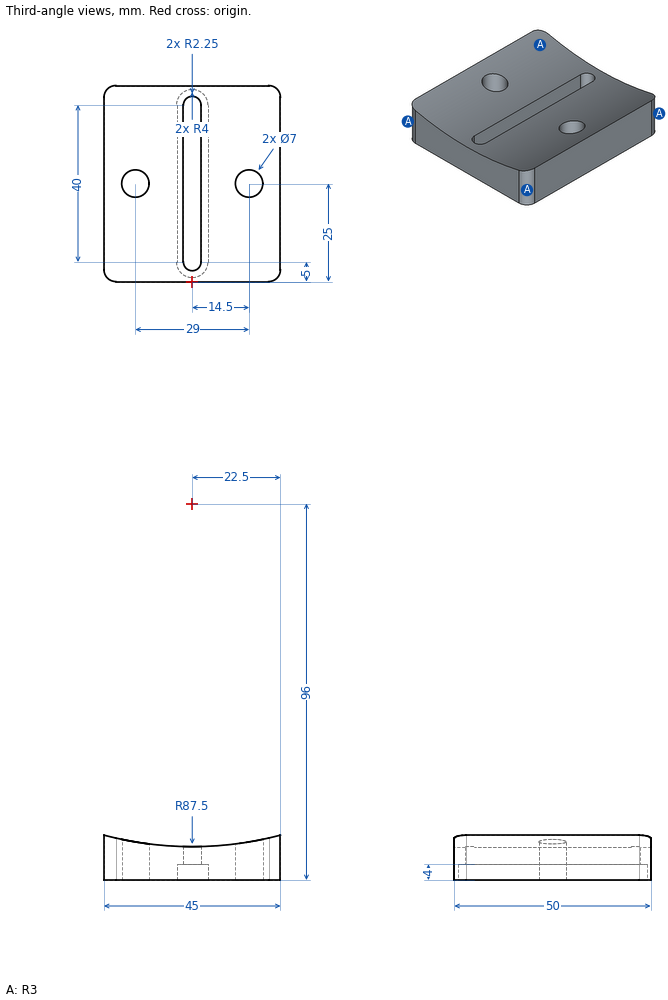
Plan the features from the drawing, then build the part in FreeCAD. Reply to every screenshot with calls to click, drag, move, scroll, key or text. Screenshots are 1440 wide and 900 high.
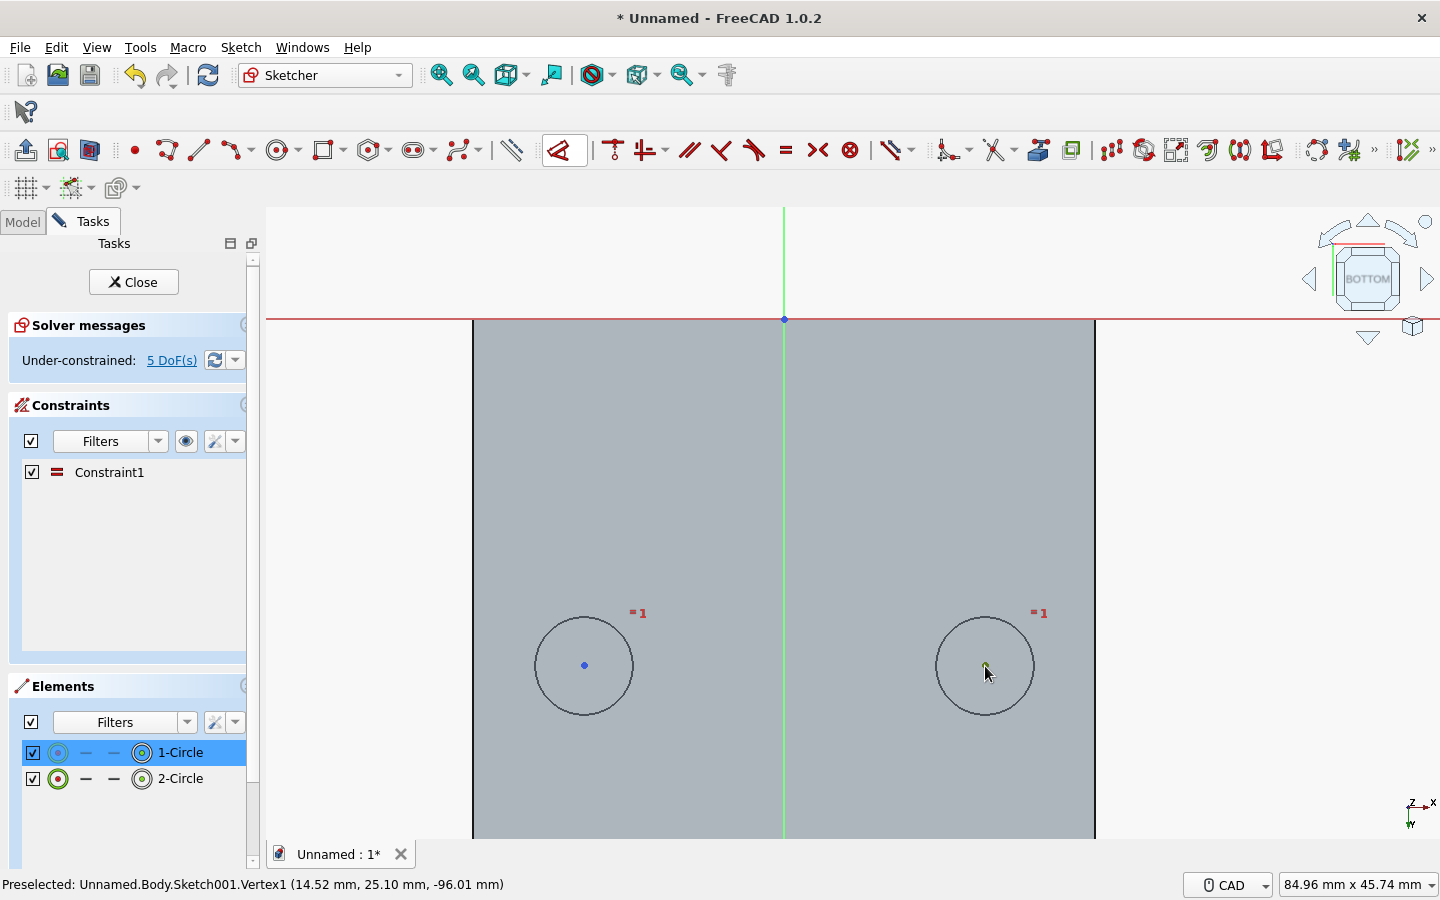
click(584, 666)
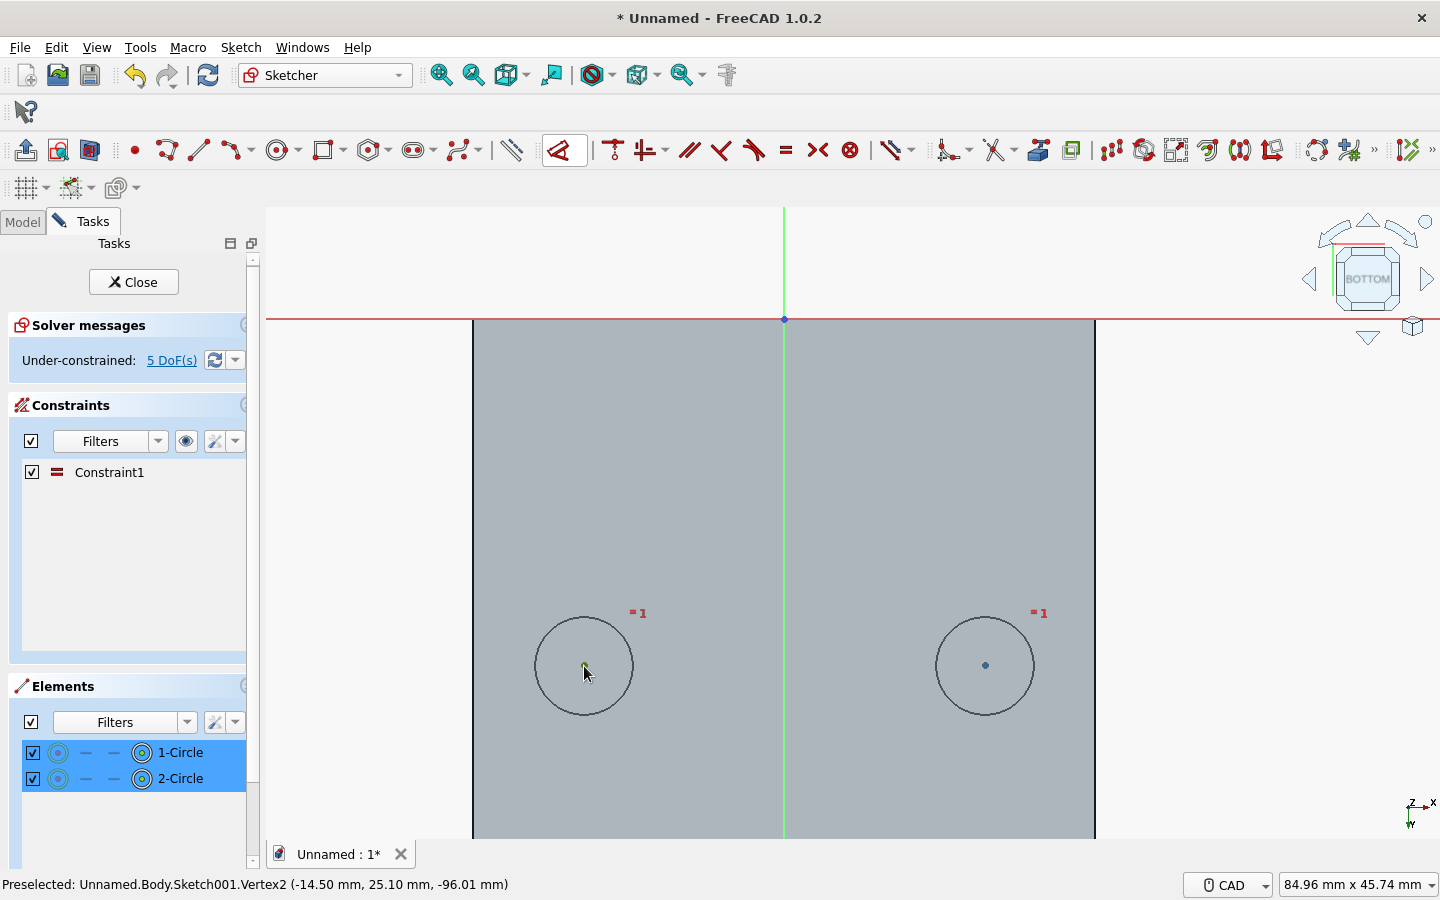
click(668, 150)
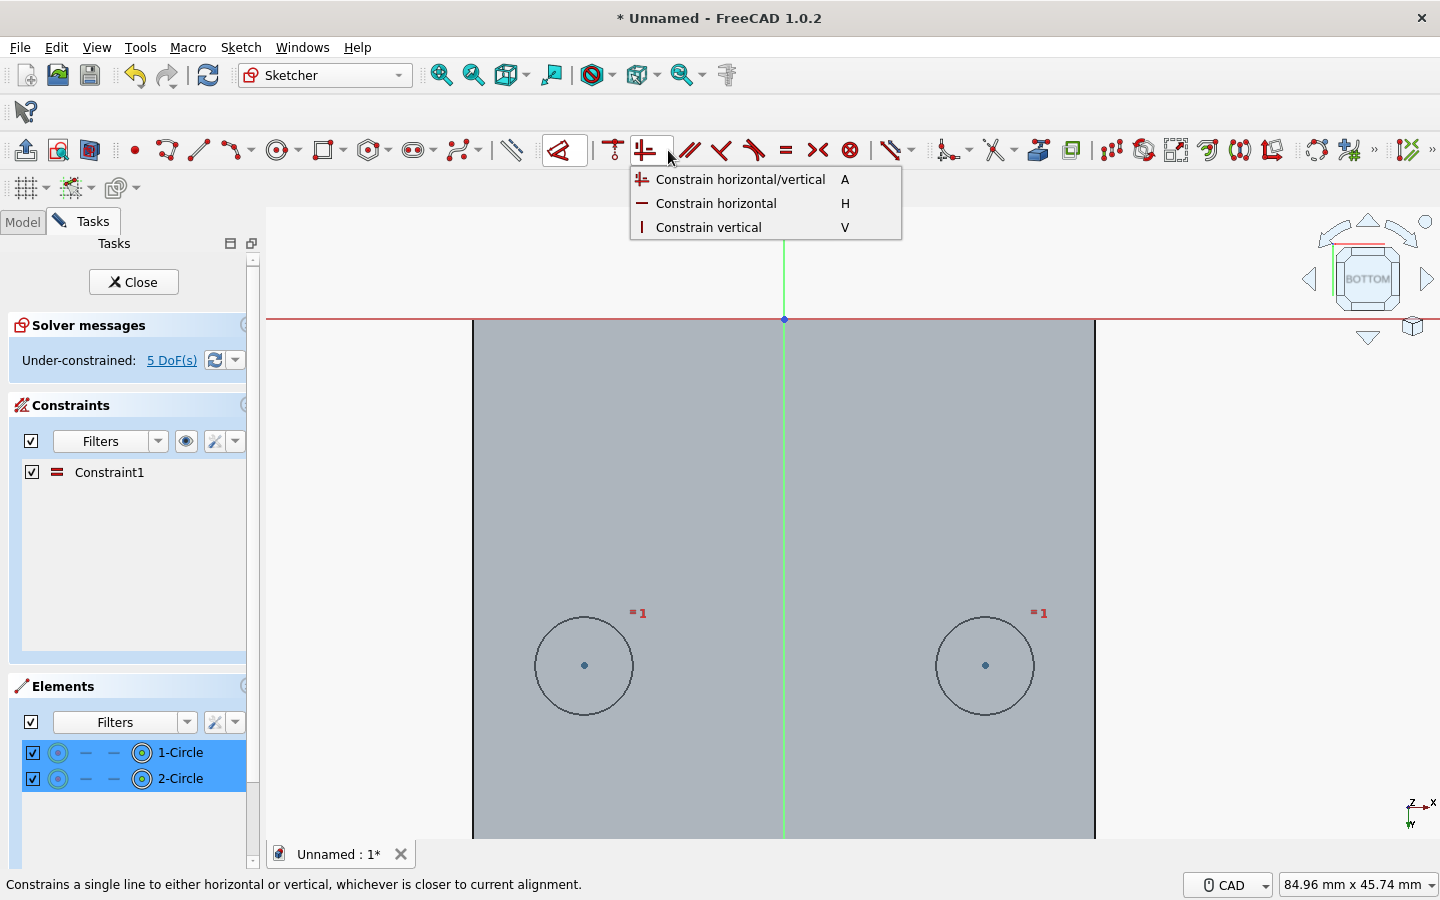
click(766, 203)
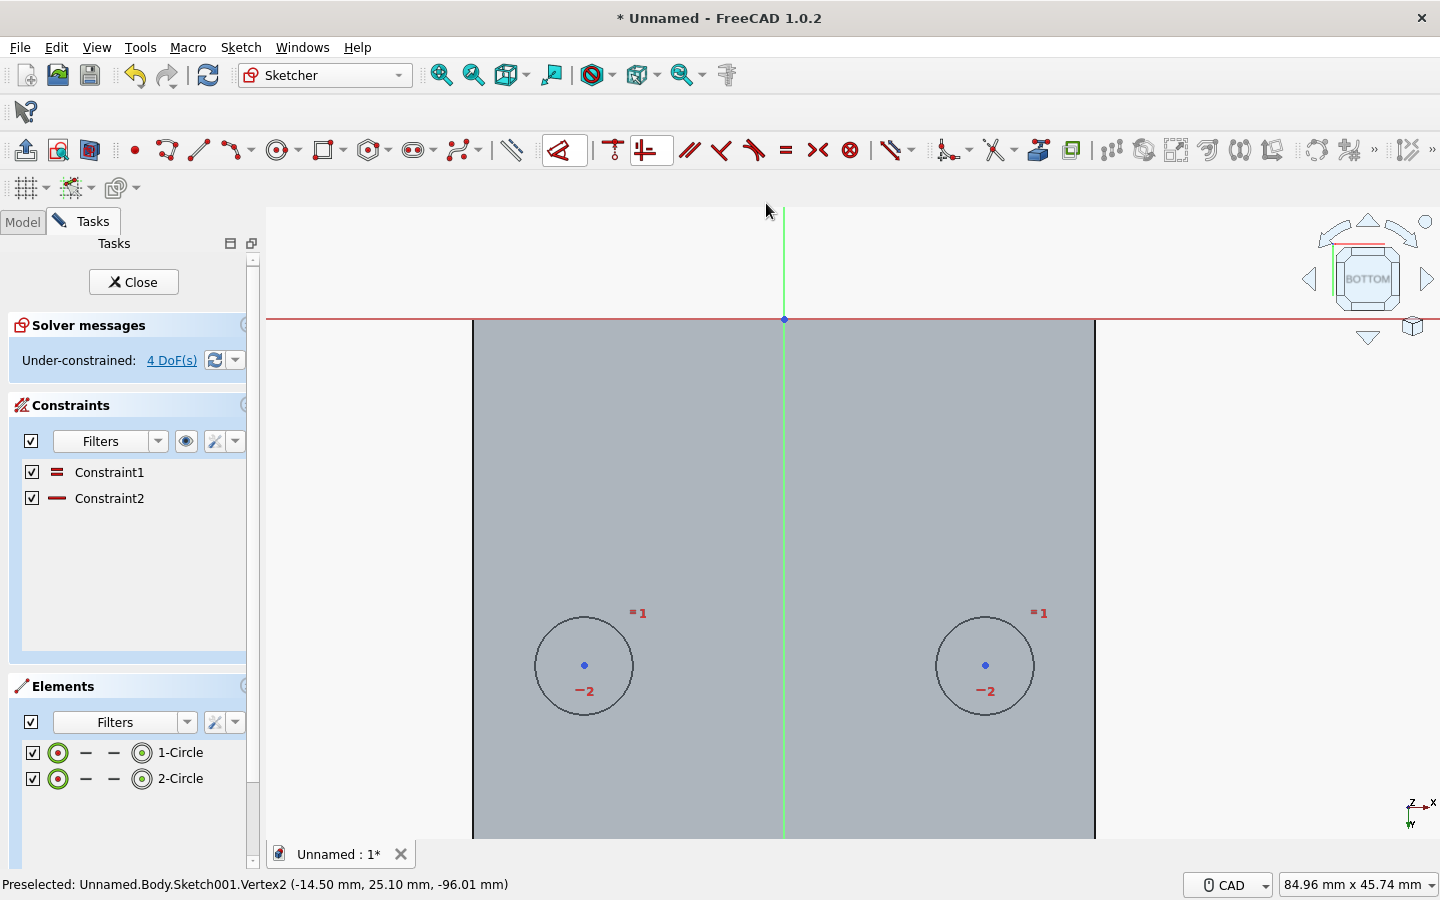
click(558, 150)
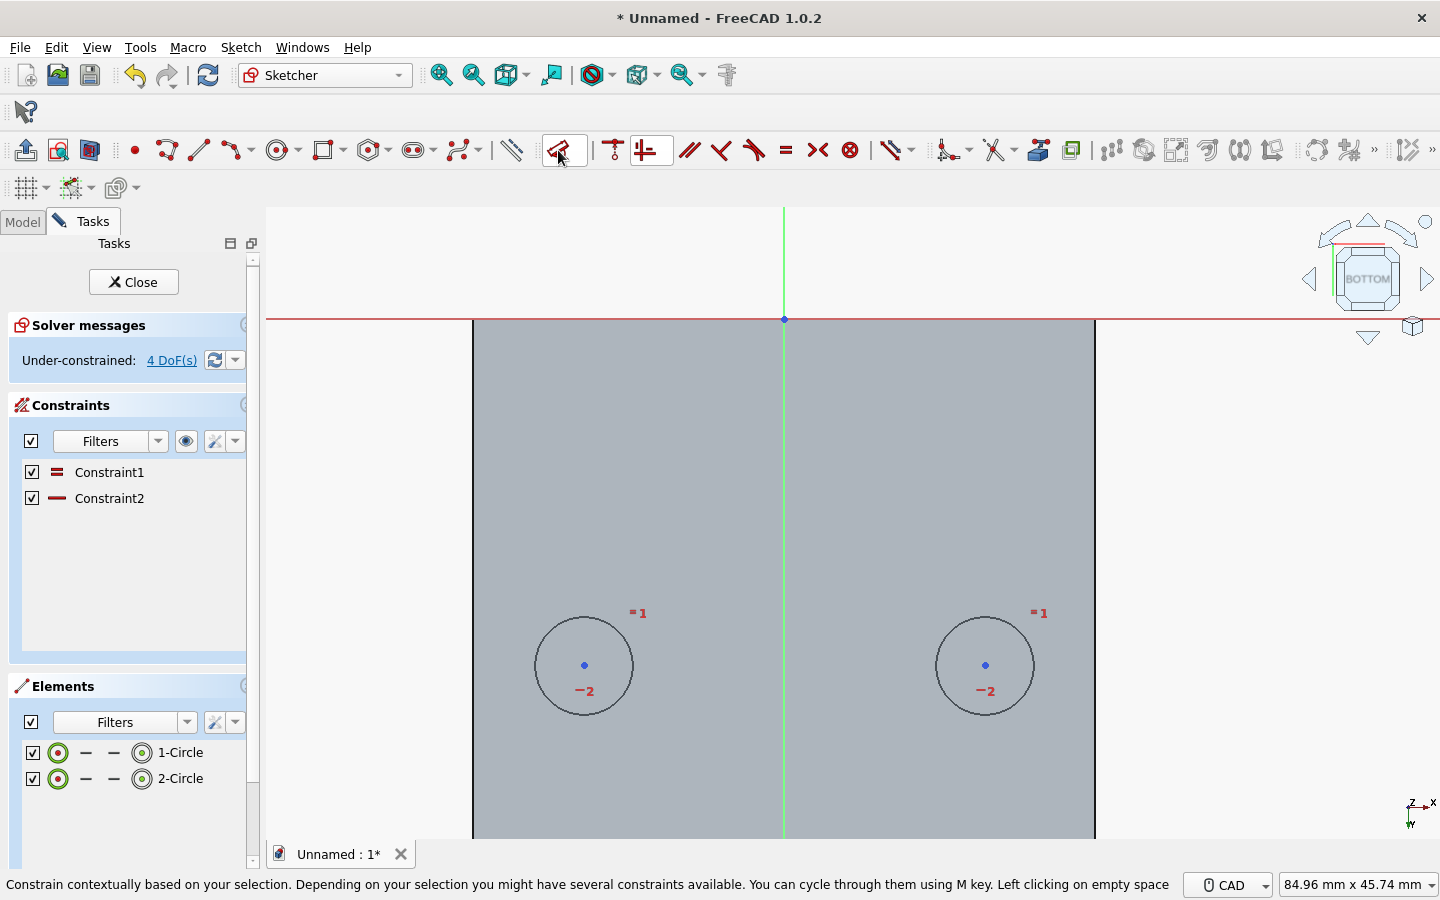
click(1019, 631)
click(1041, 608)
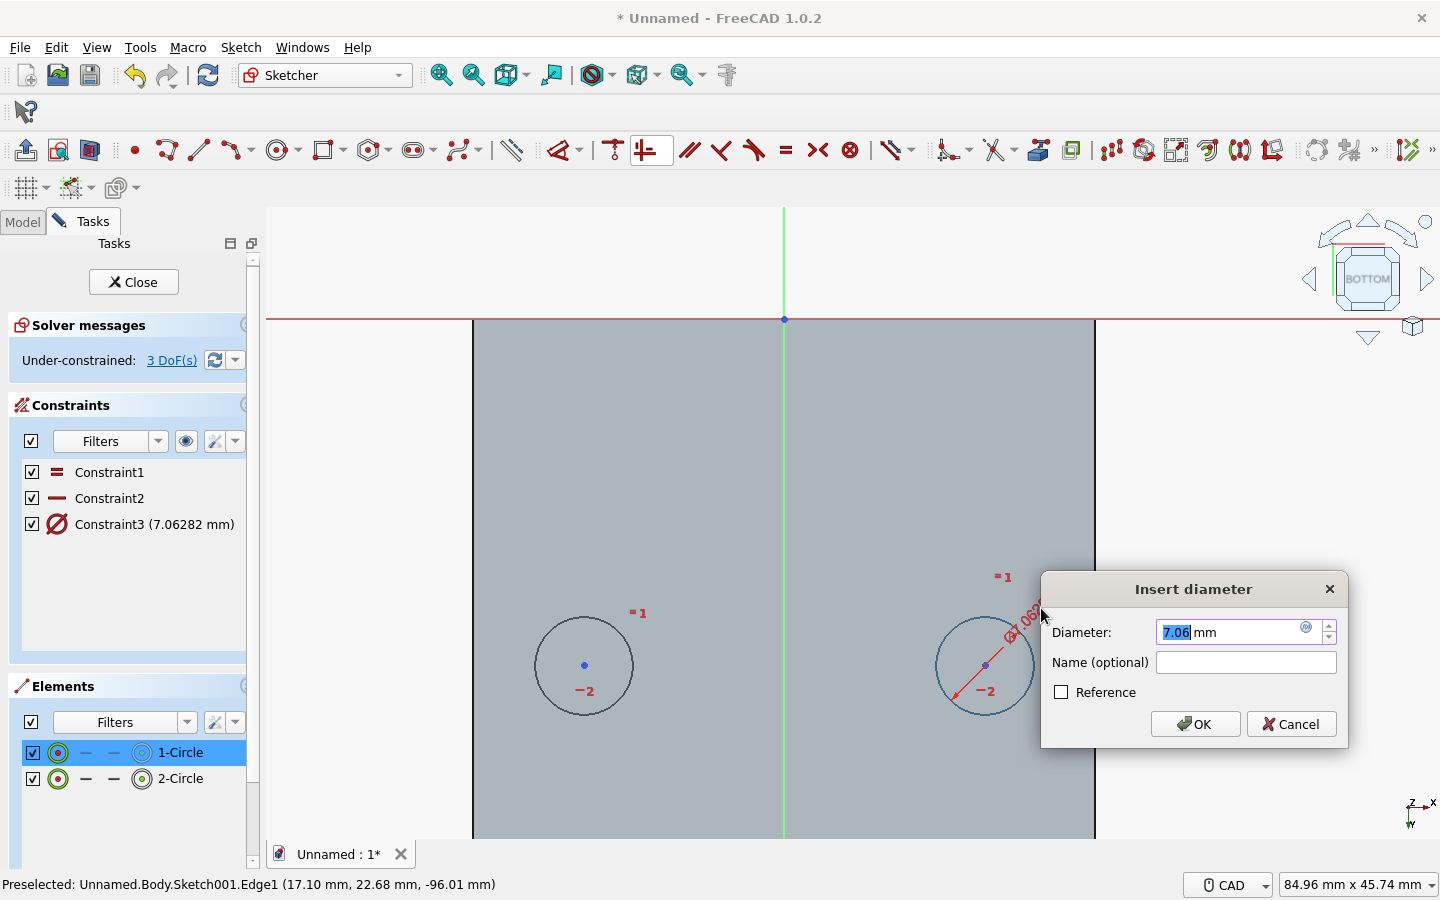
text(7)
key(Return)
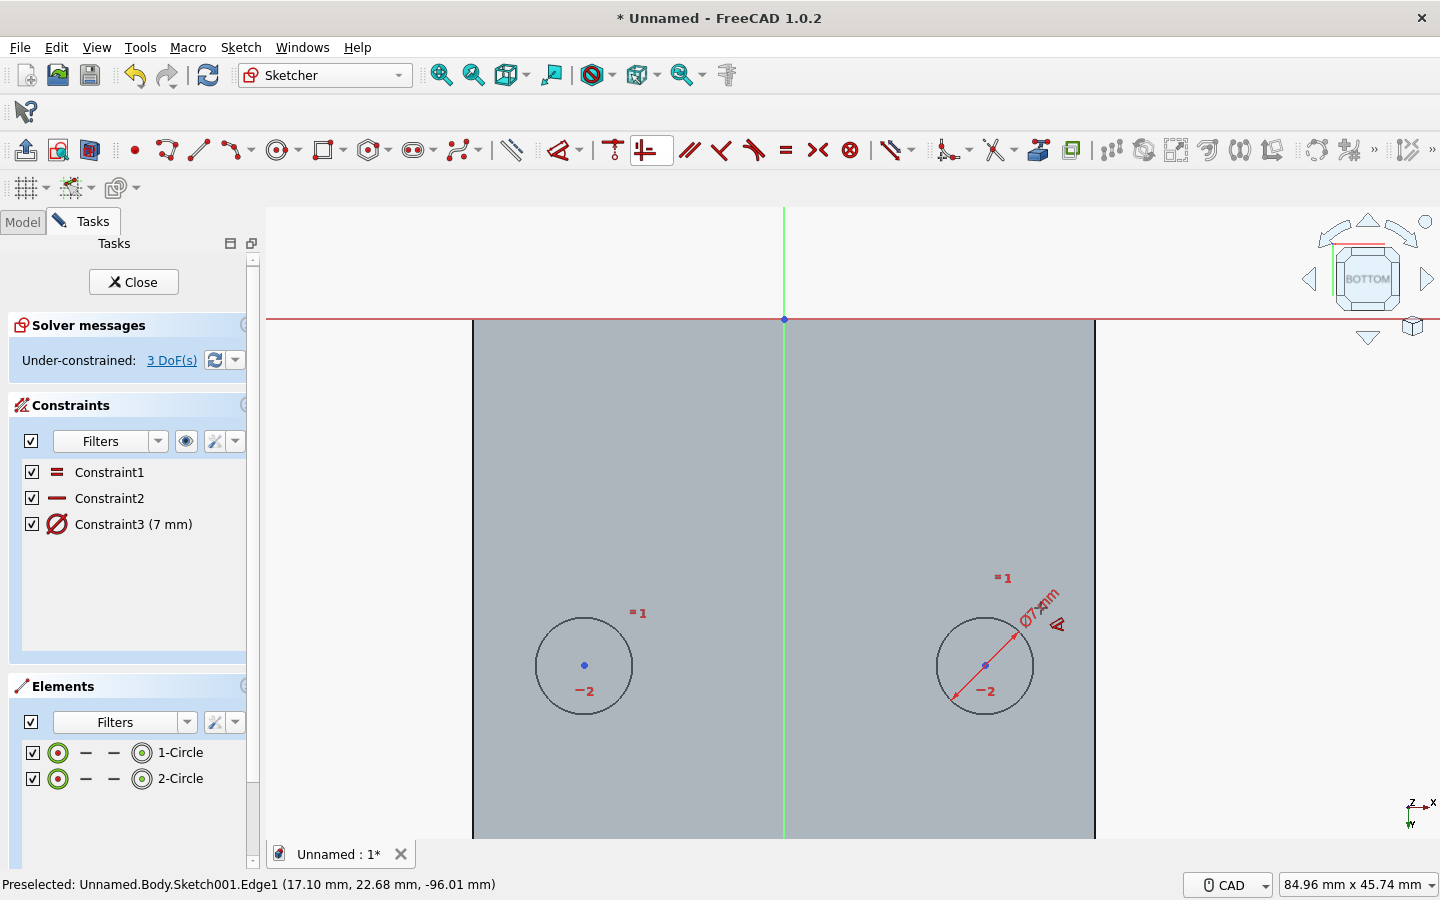
click(985, 666)
click(1019, 493)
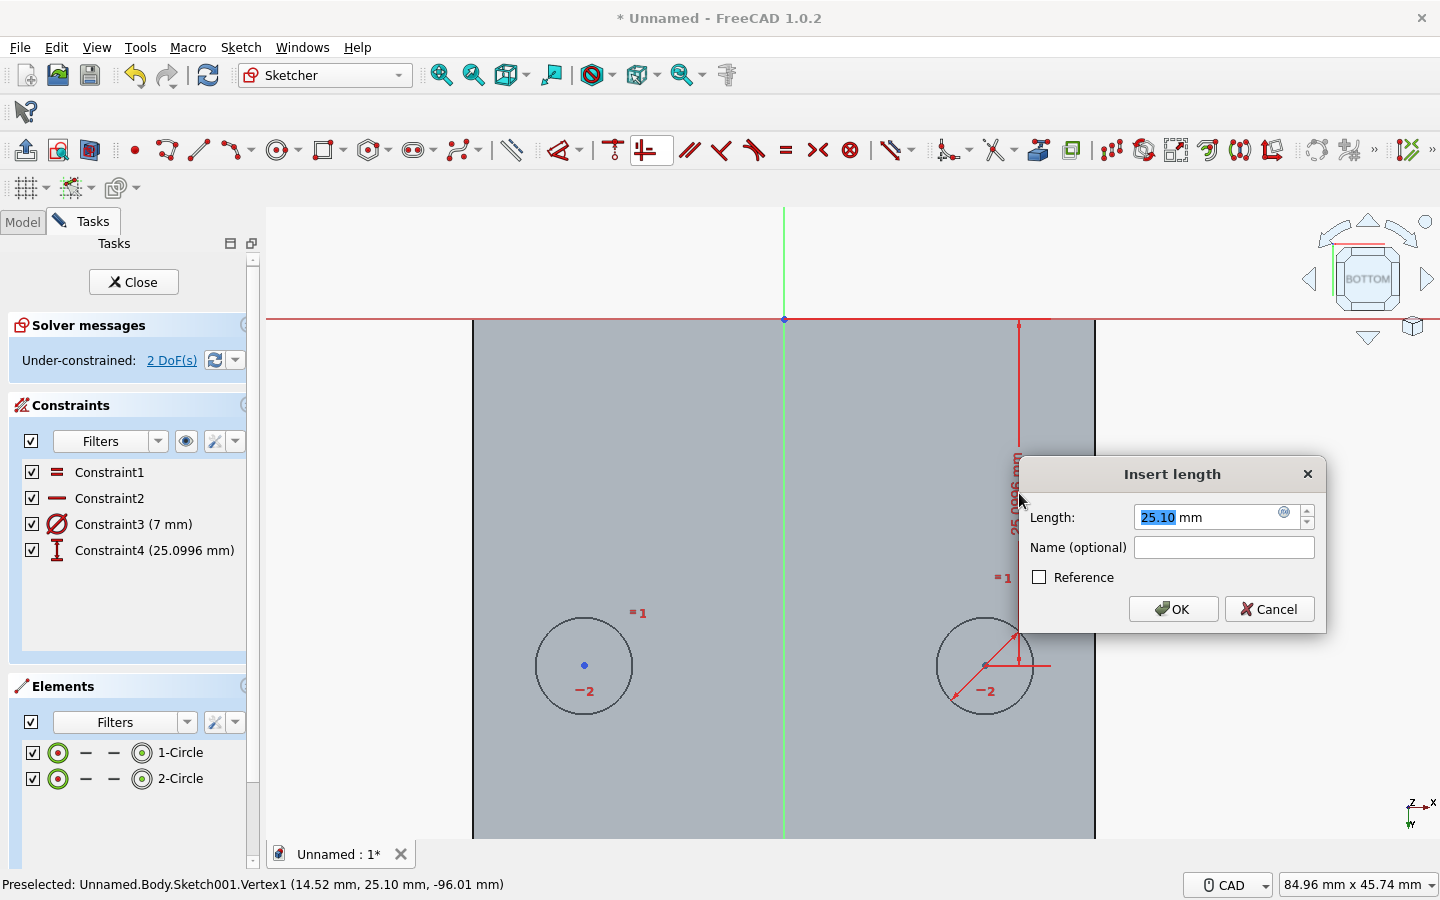
text(25)
key(Return)